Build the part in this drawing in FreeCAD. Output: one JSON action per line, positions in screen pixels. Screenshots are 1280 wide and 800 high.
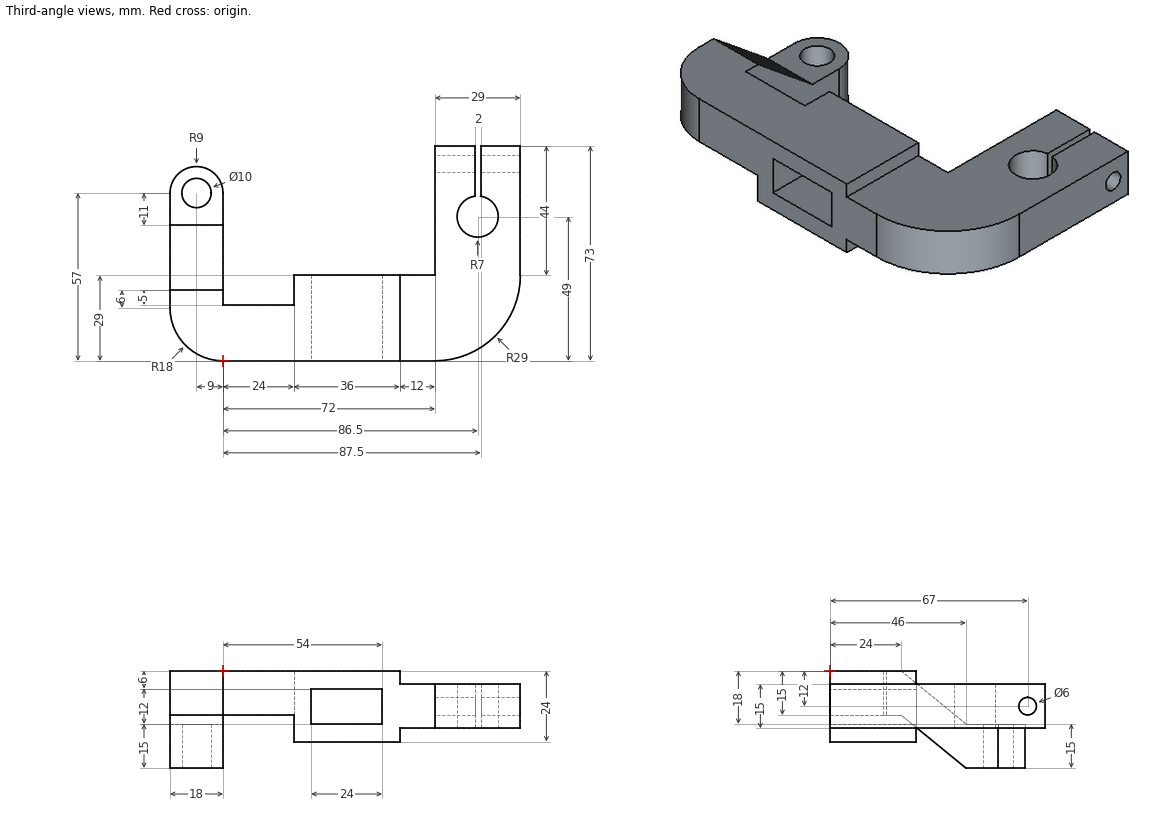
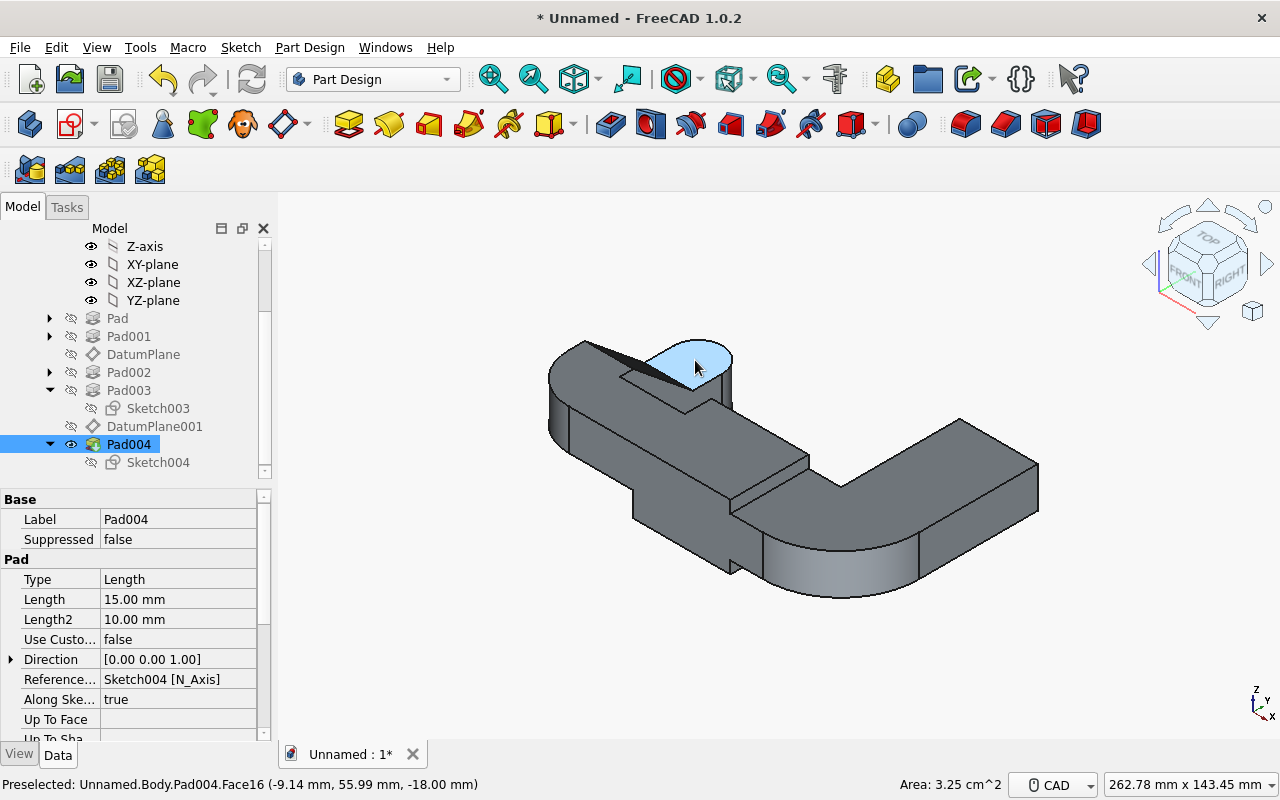
{"action": "left_click", "coordinate": [70, 124]}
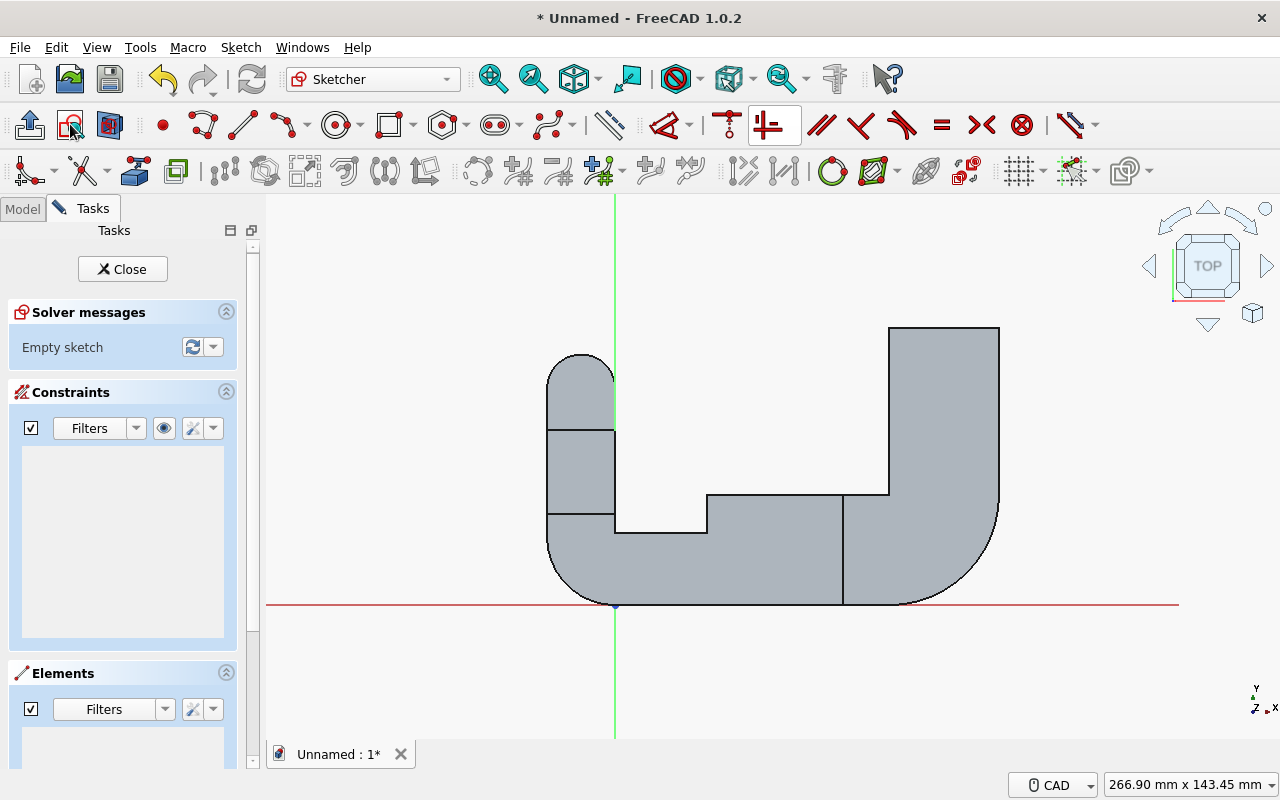
{"action": "scroll", "coordinate": [566, 379], "scroll_direction": "up", "scroll_amount": 11}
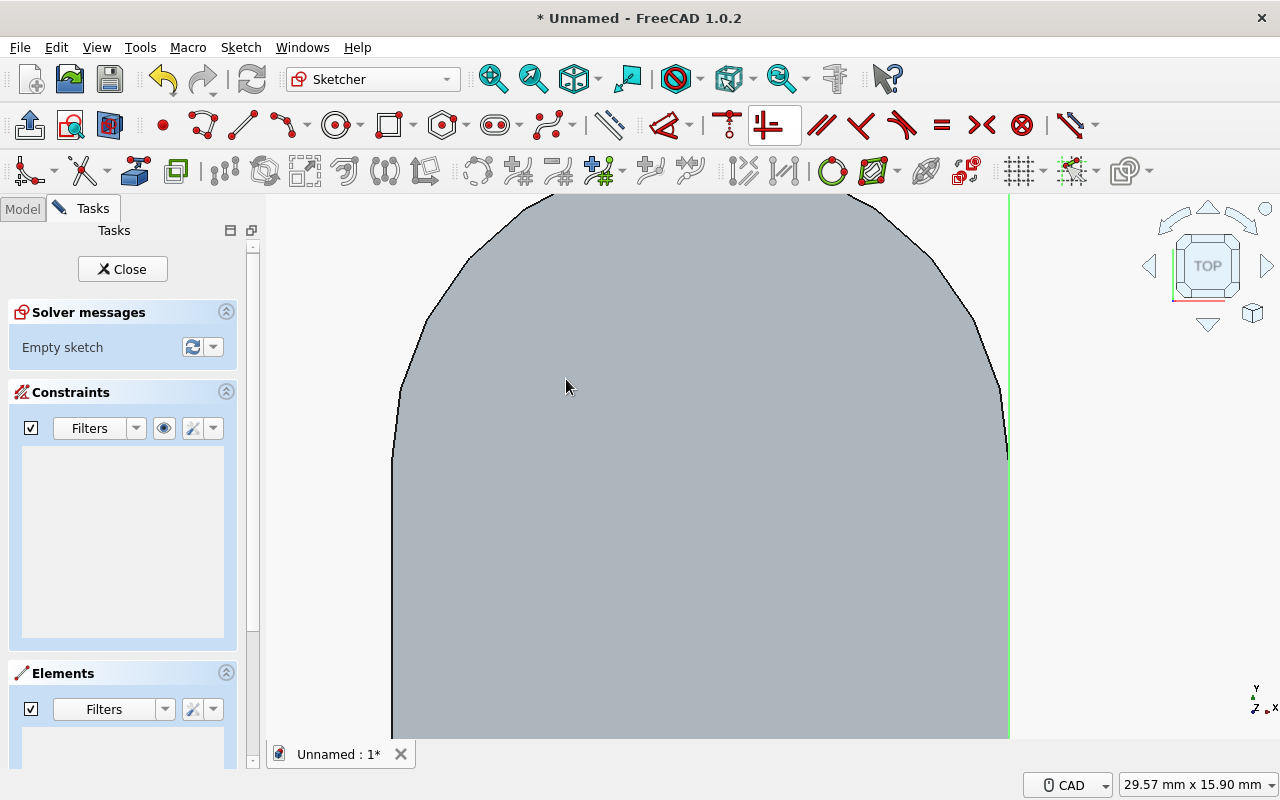
{"action": "left_click", "coordinate": [336, 126]}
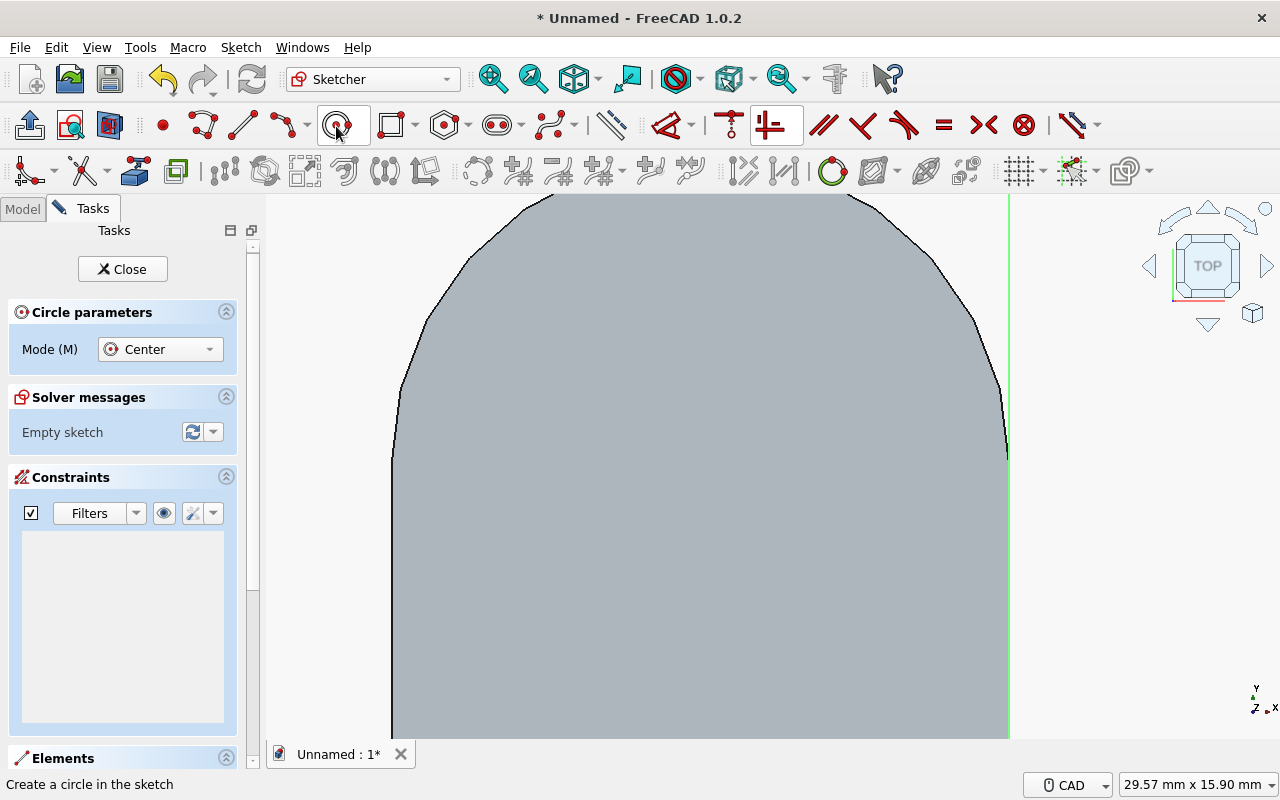
{"action": "left_click", "coordinate": [700, 463]}
{"action": "mouse_move", "coordinate": [822, 342]}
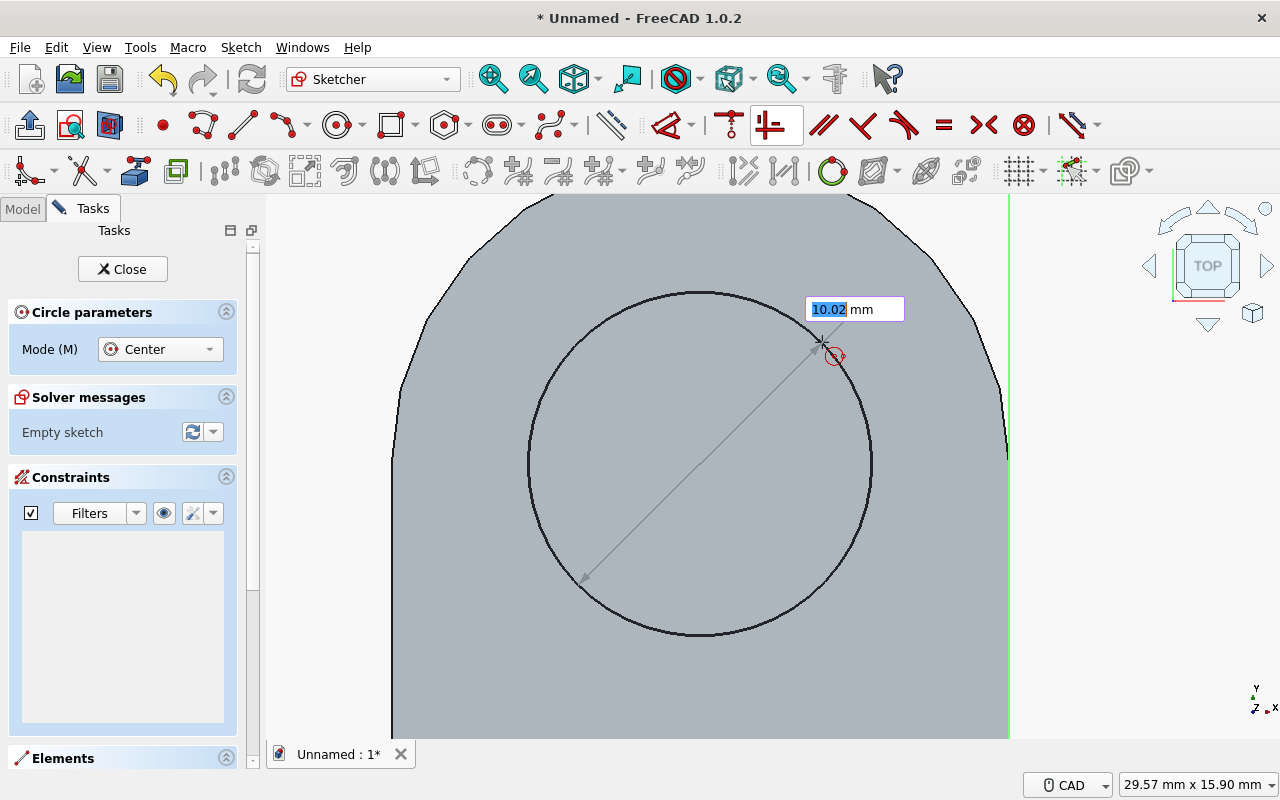
{"action": "type", "text": "10"}
{"action": "key", "text": "Return"}
{"action": "key", "text": "Escape"}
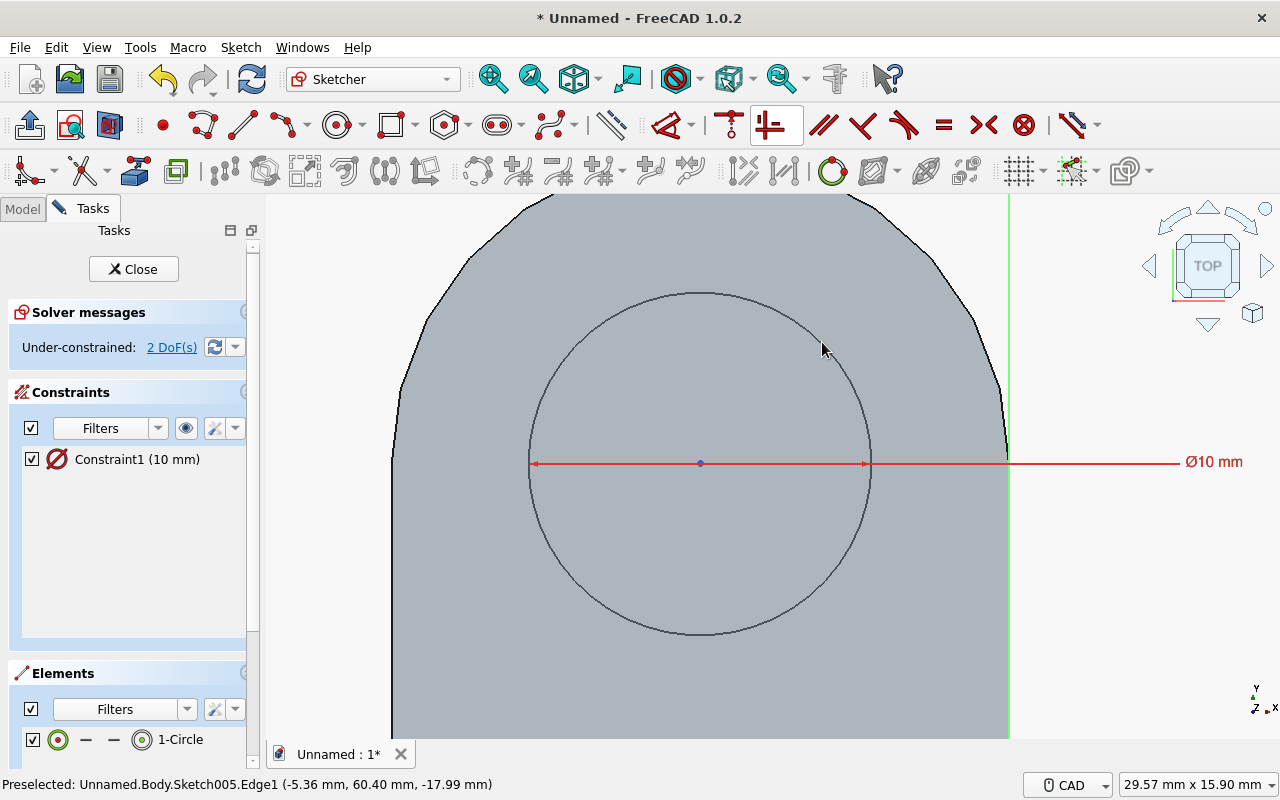
{"action": "left_click", "coordinate": [666, 126]}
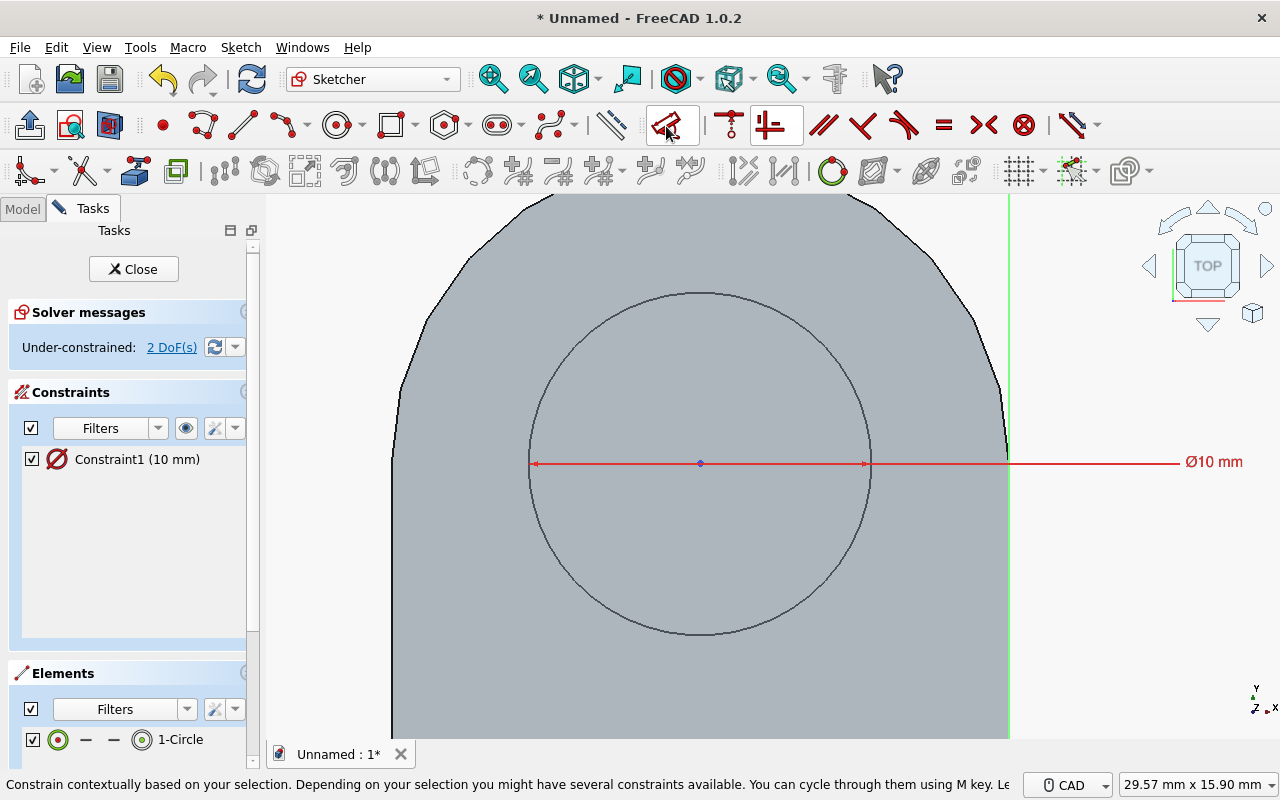
{"action": "left_click", "coordinate": [700, 464]}
{"action": "left_click", "coordinate": [854, 430]}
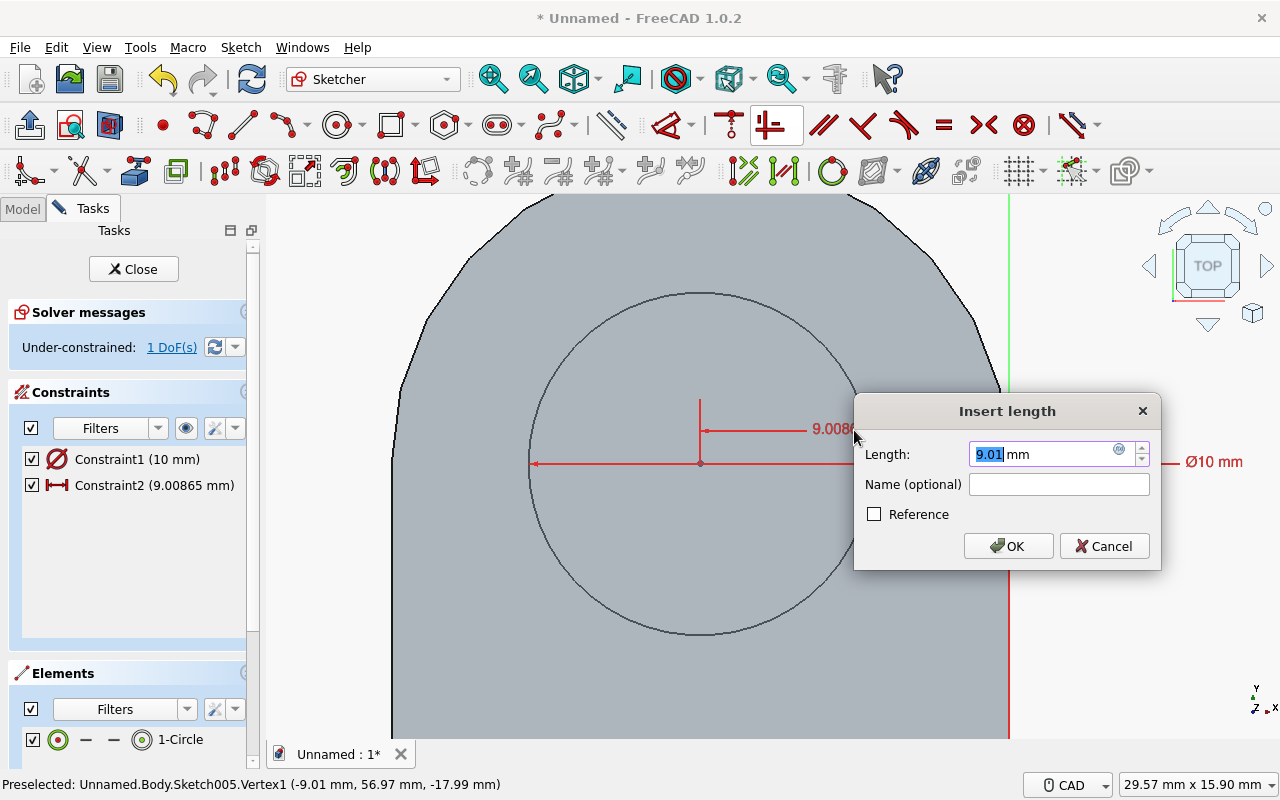
{"action": "type", "text": "9"}
{"action": "key", "text": "Return"}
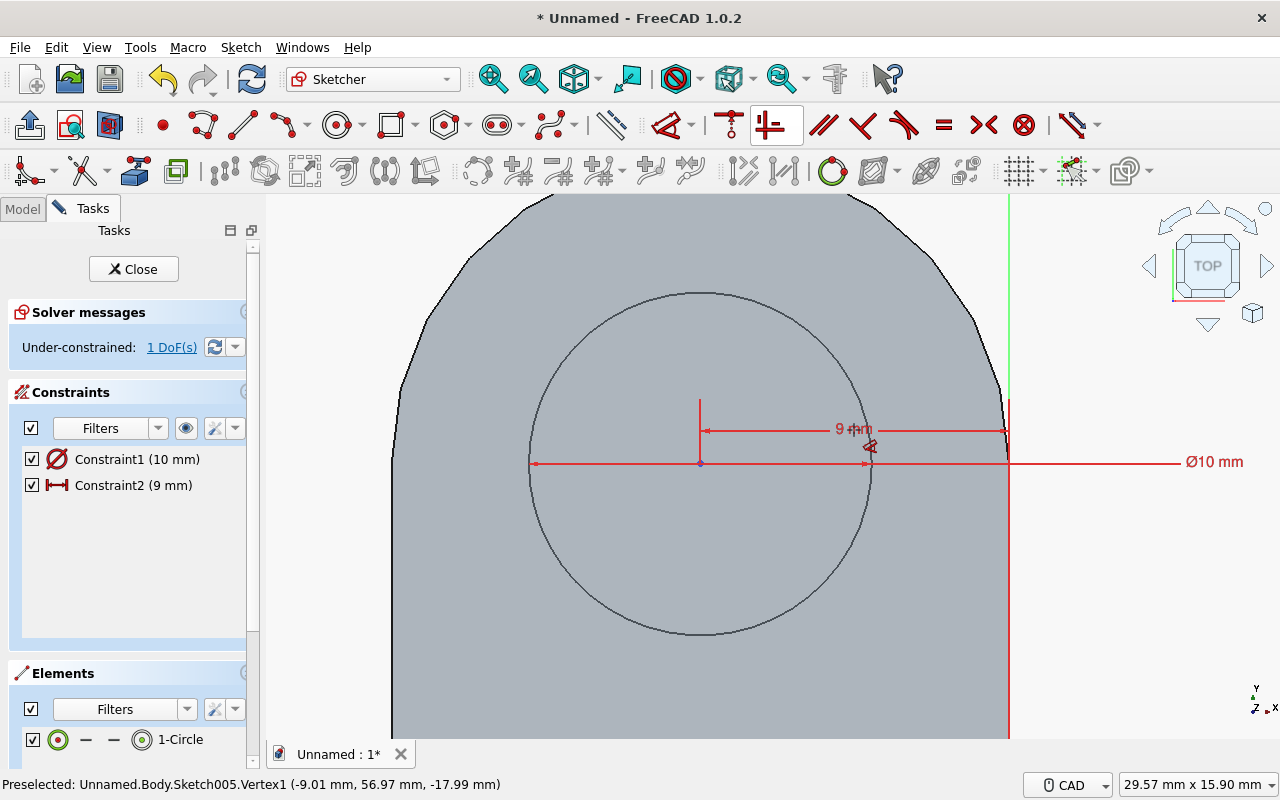
{"action": "left_click", "coordinate": [700, 464]}
{"action": "left_click", "coordinate": [1043, 587]}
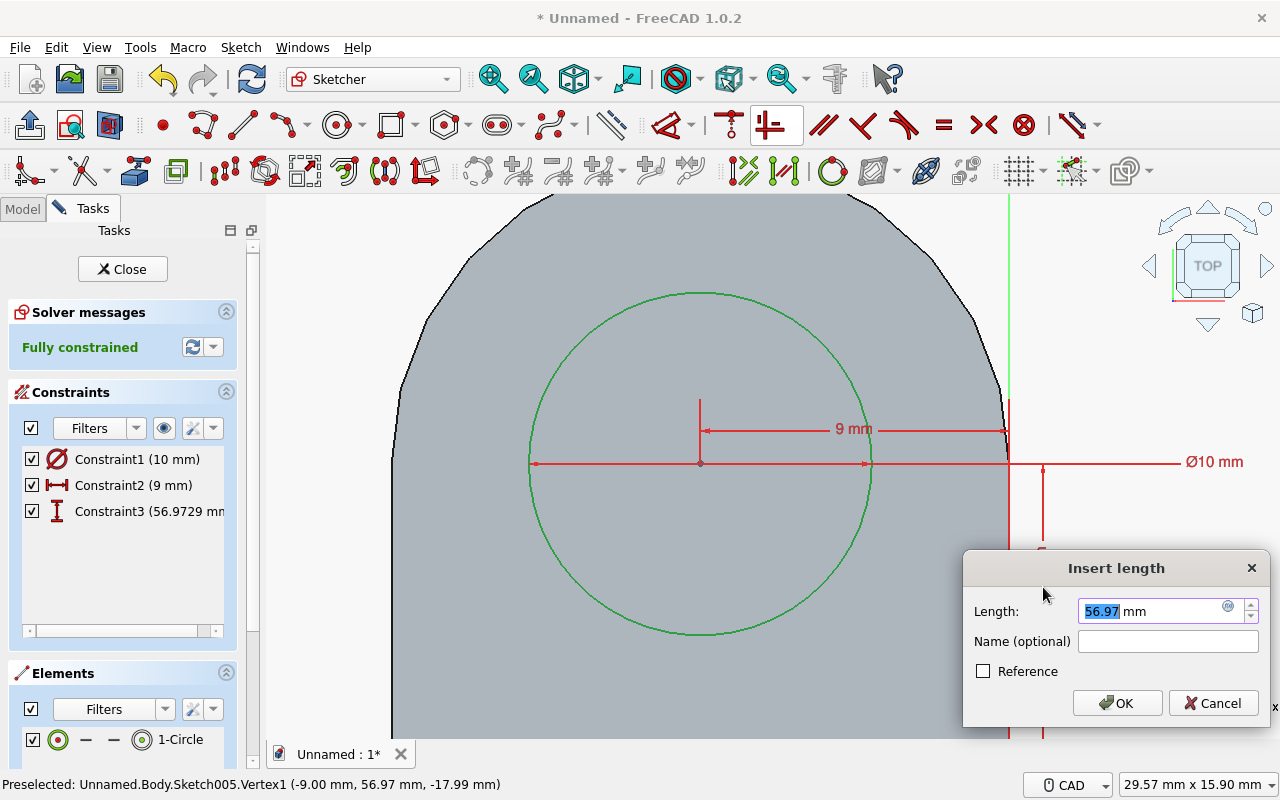
{"action": "type", "text": "57"}
{"action": "key", "text": "Return"}
{"action": "key", "text": "Escape"}